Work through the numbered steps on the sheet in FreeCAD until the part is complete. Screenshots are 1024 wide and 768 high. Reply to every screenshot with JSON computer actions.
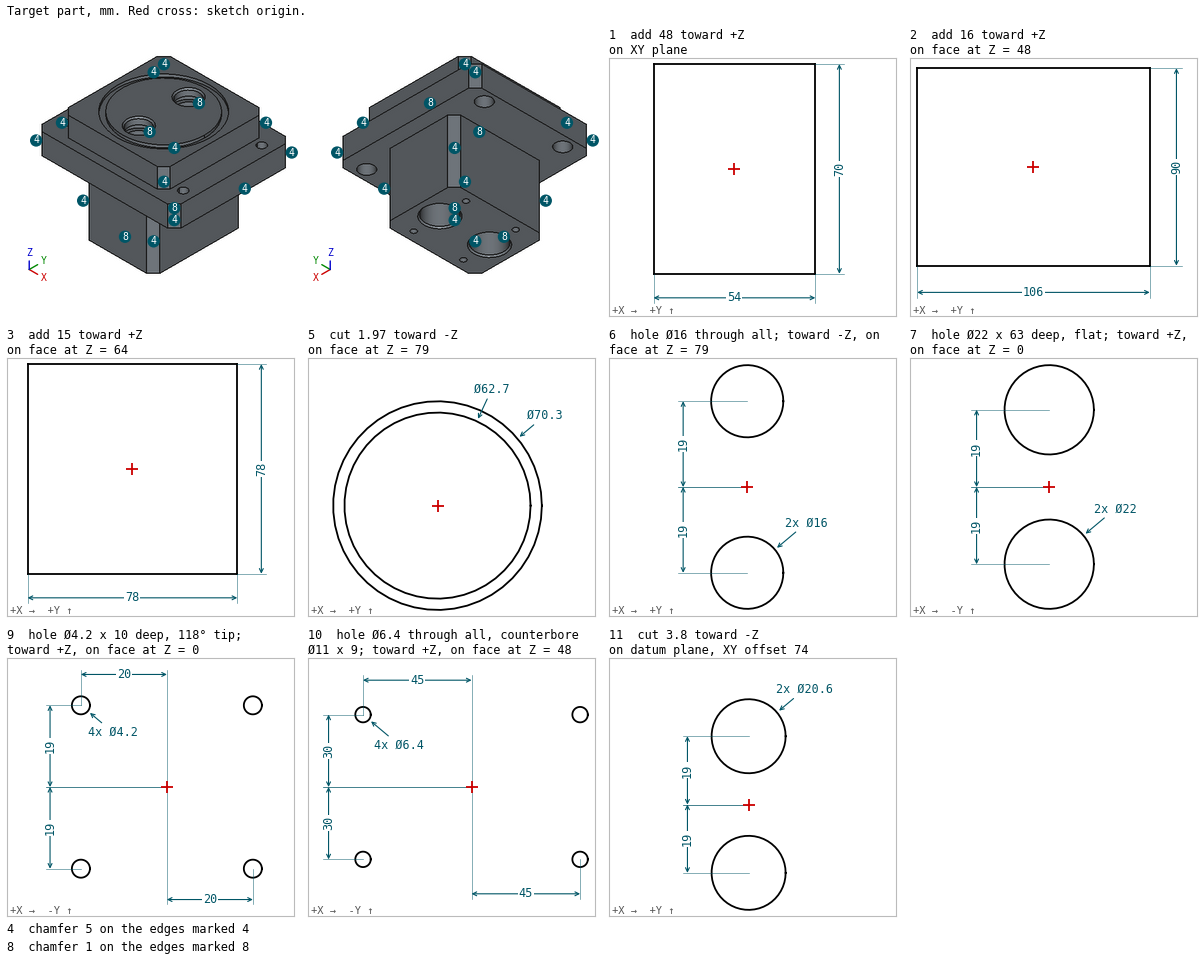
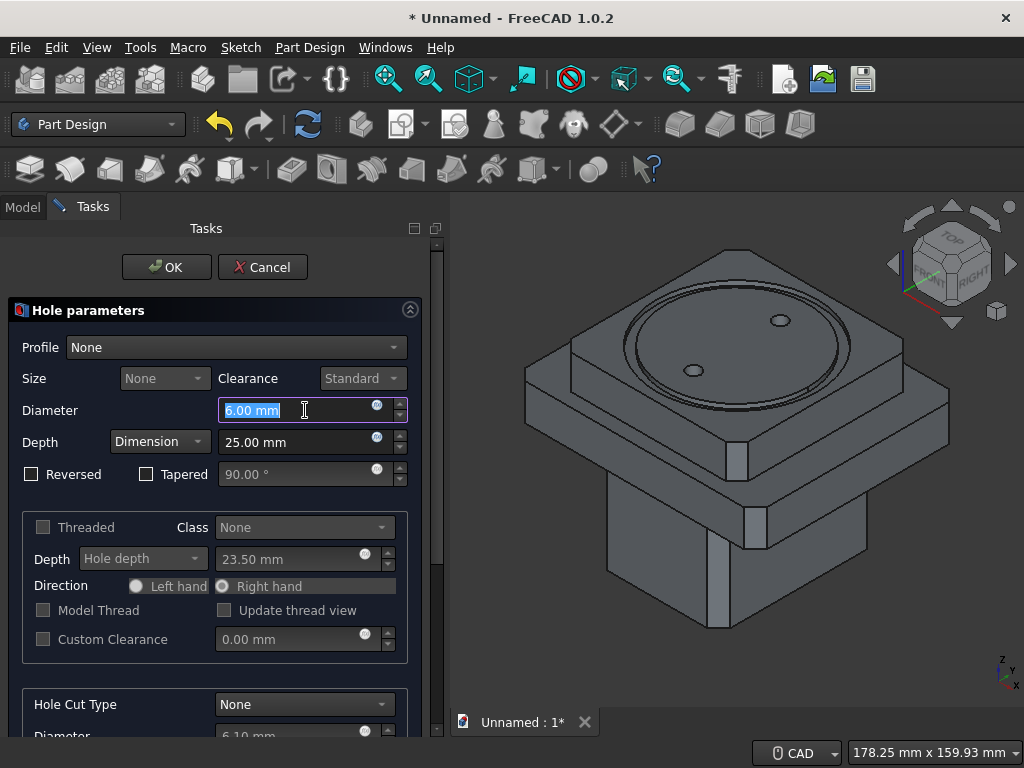
{"action": "type", "text": "16"}
{"action": "key", "text": "Tab"}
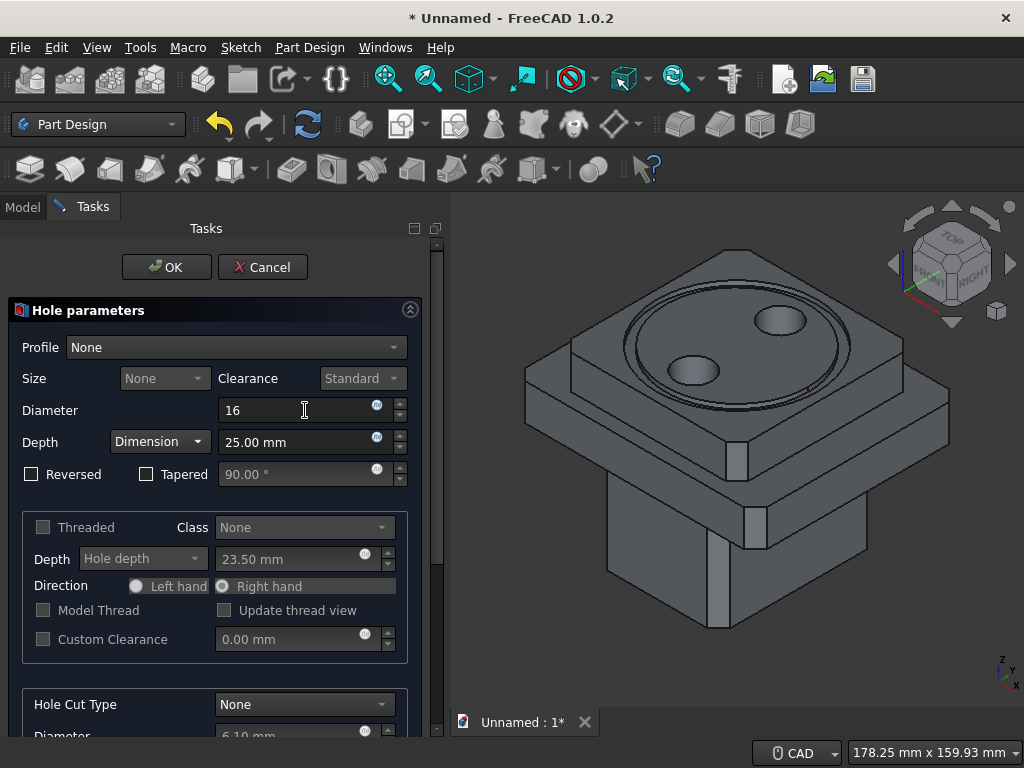
{"action": "left_click", "coordinate": [161, 442]}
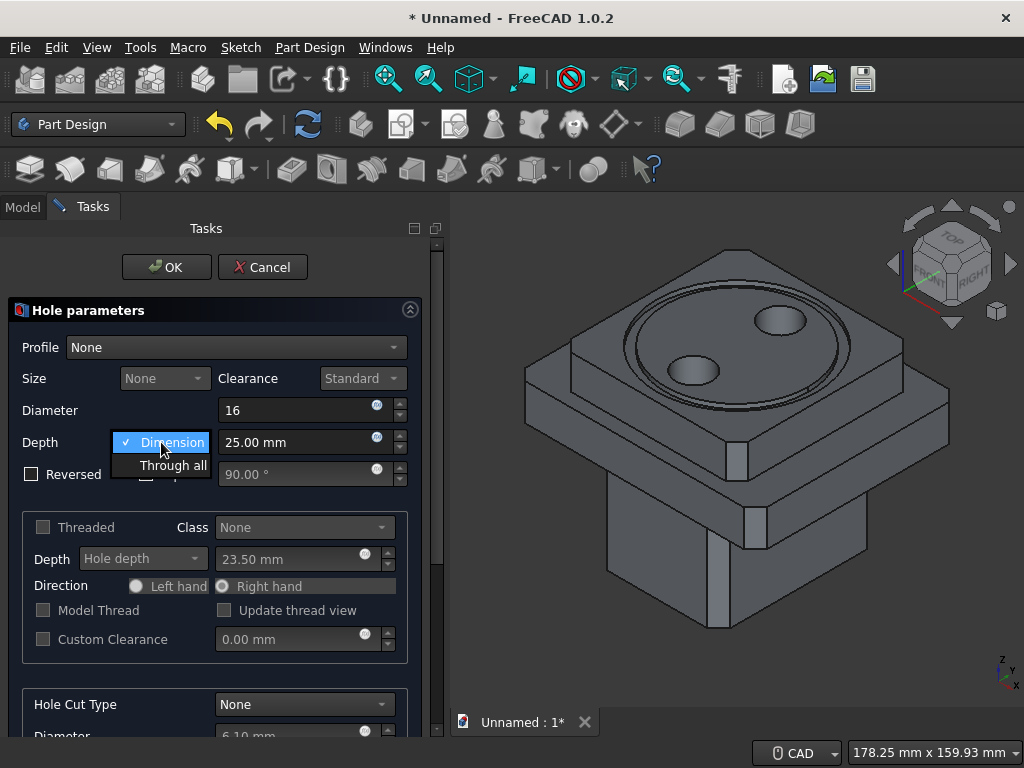
{"action": "left_click", "coordinate": [160, 466]}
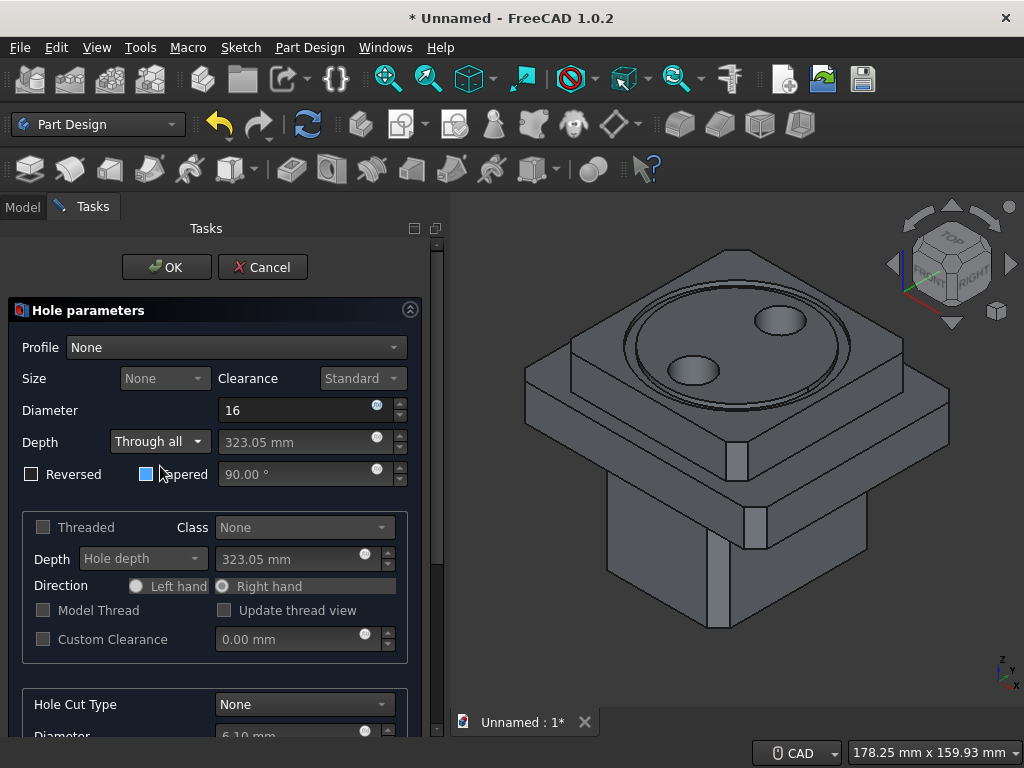
{"action": "left_click", "coordinate": [167, 267]}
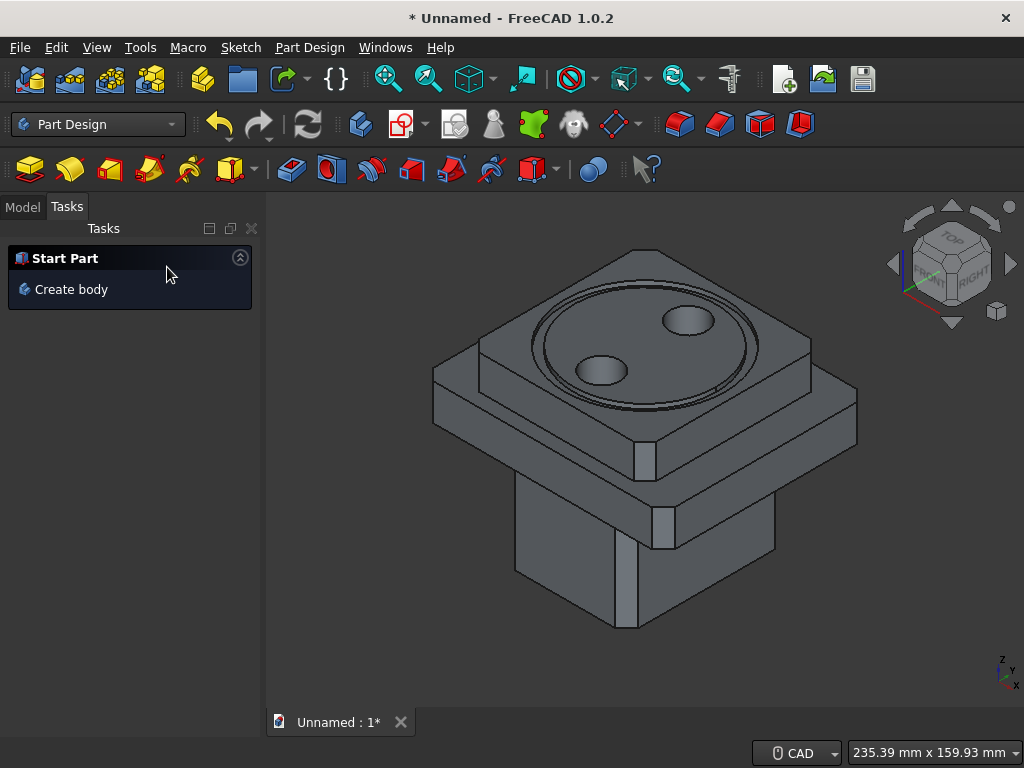
{"action": "key", "text": "5"}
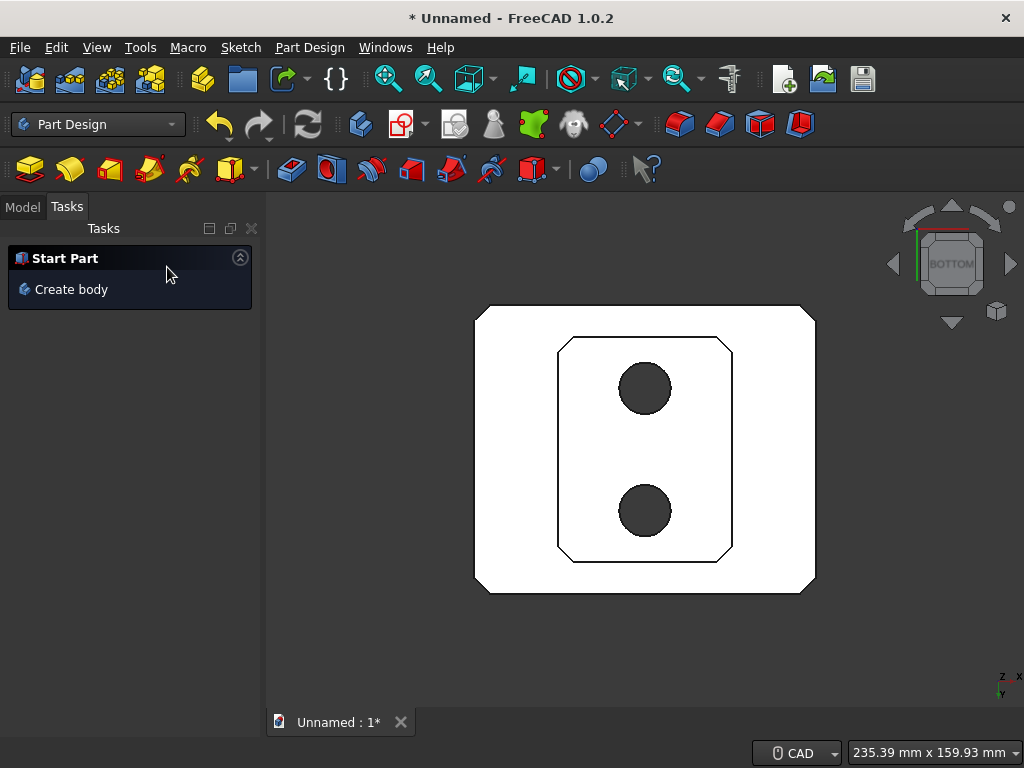
{"action": "left_click", "coordinate": [670, 449]}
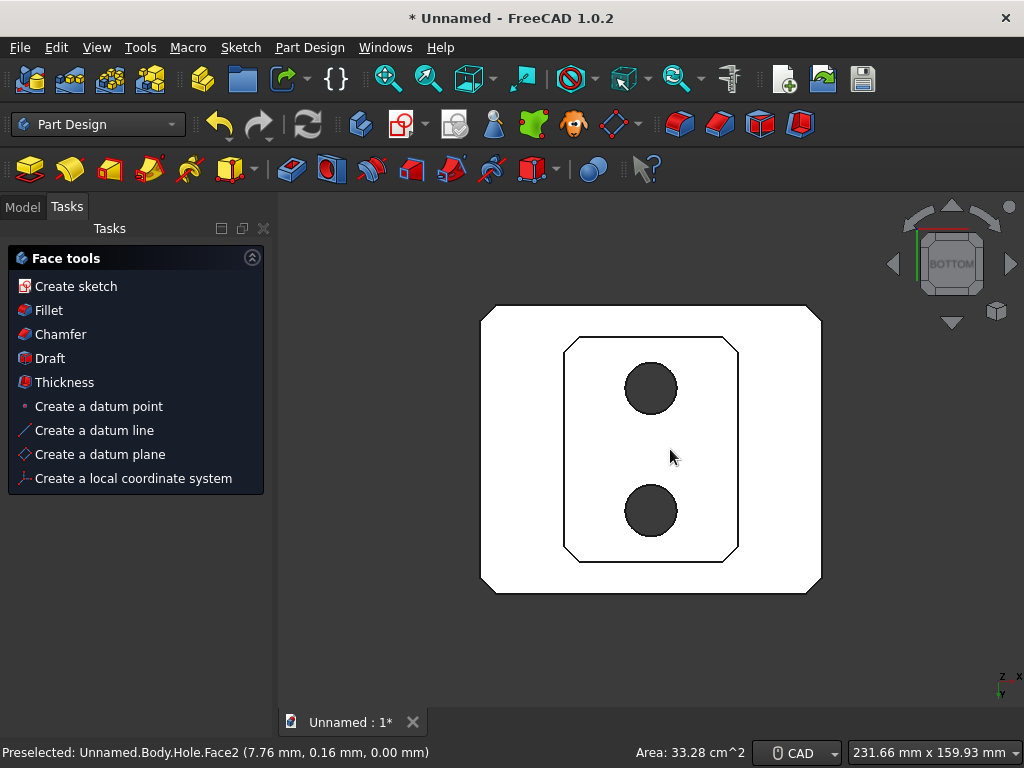
{"action": "left_click", "coordinate": [402, 124]}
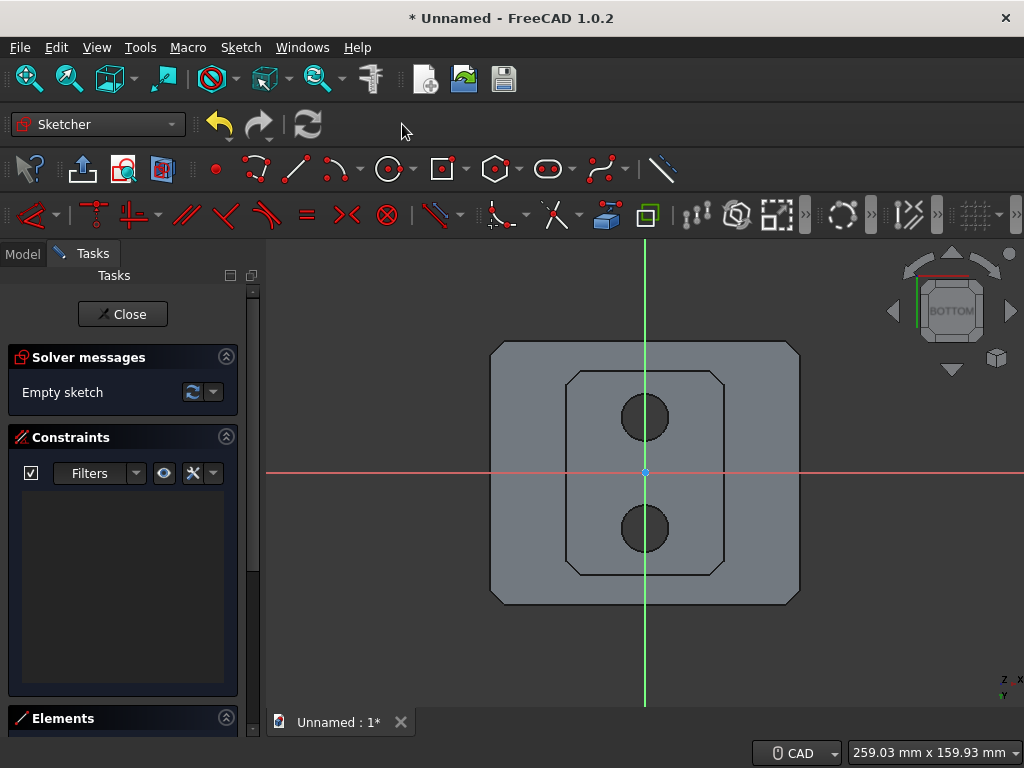
{"action": "scroll", "coordinate": [728, 473], "scroll_direction": "up", "scroll_amount": 3}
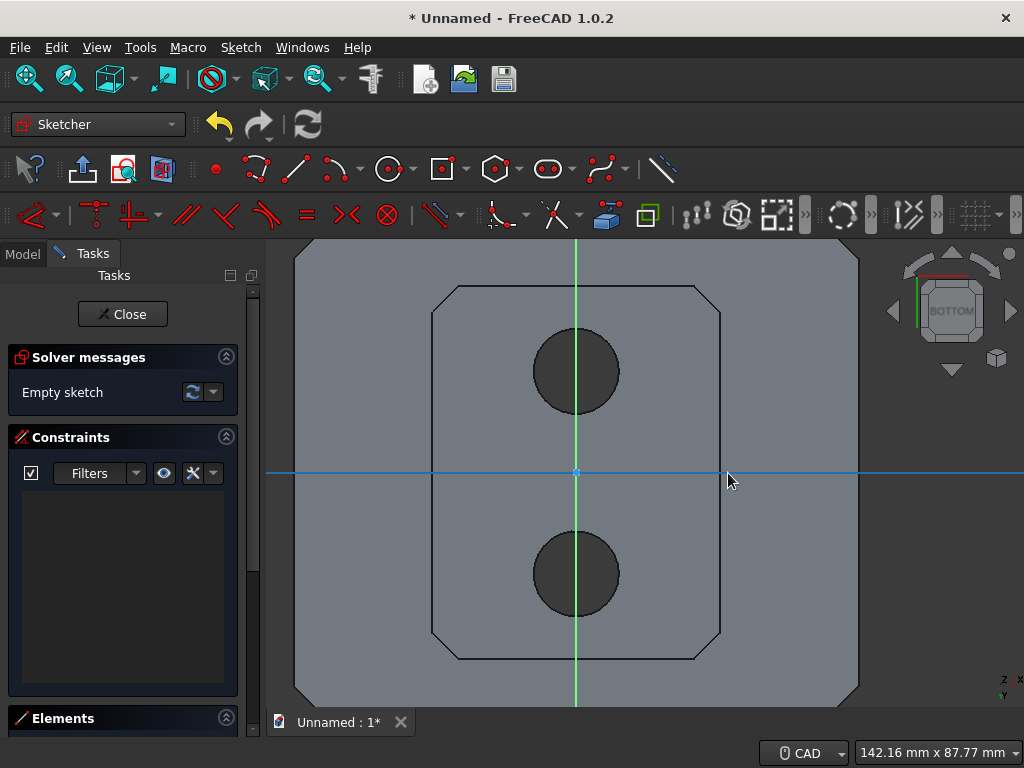
{"action": "left_click", "coordinate": [390, 170]}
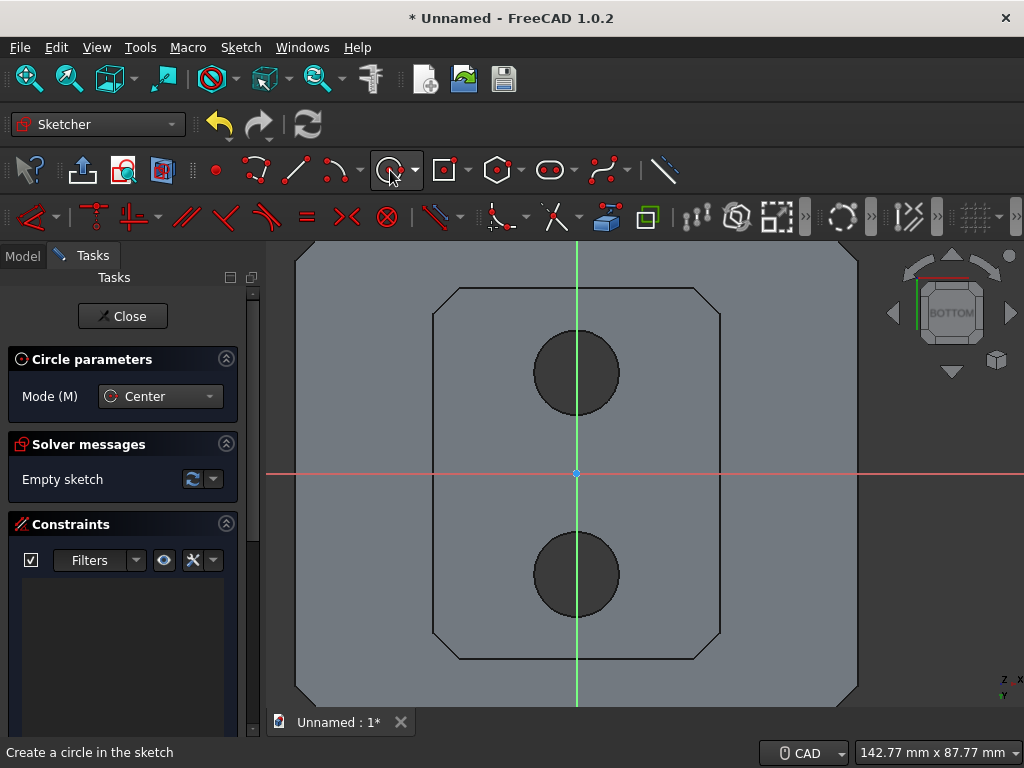
{"action": "left_click", "coordinate": [577, 574]}
{"action": "mouse_move", "coordinate": [618, 533]}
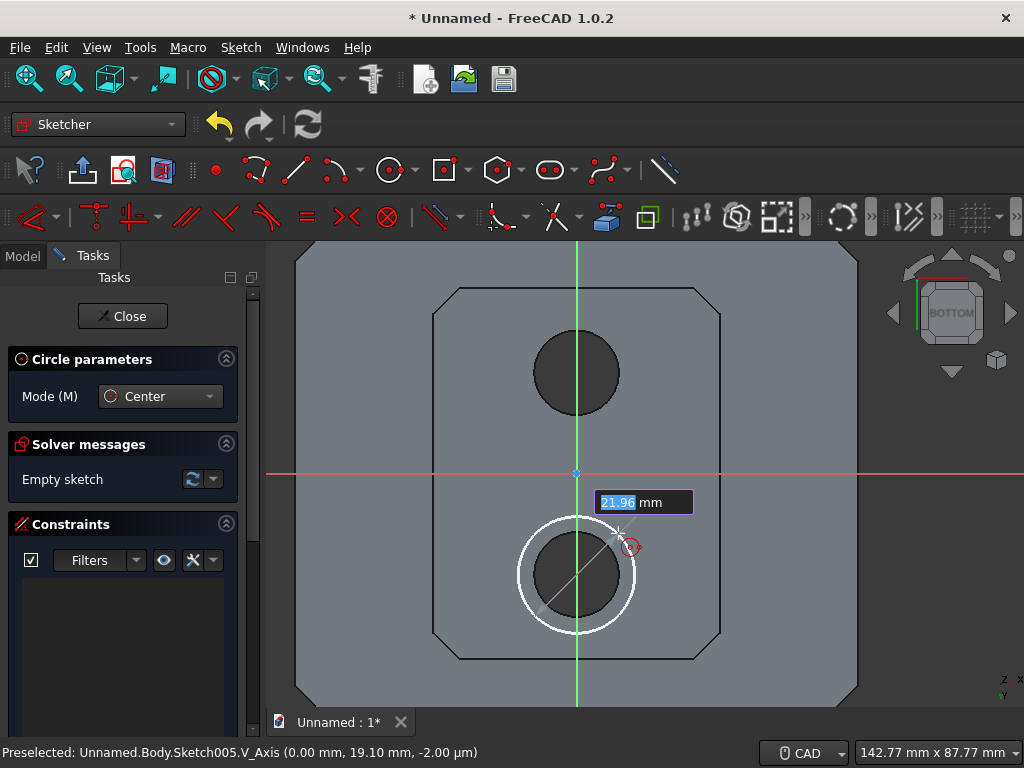
{"action": "type", "text": "22"}
{"action": "key", "text": "Return"}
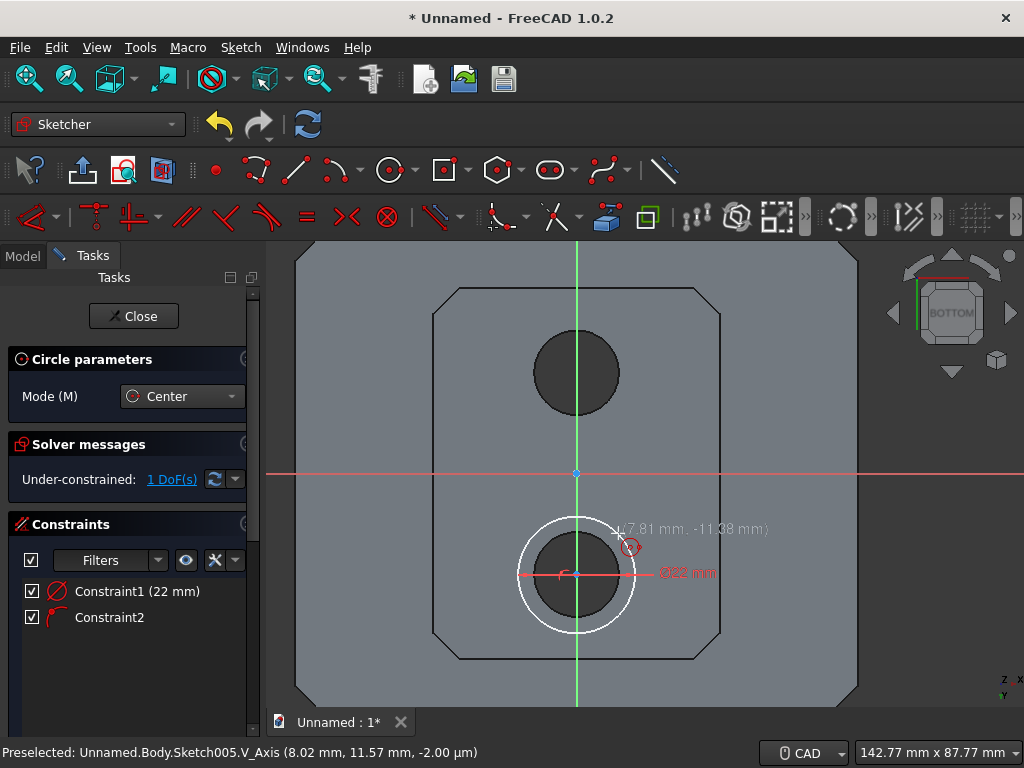
{"action": "left_click", "coordinate": [577, 373]}
{"action": "mouse_move", "coordinate": [618, 331]}